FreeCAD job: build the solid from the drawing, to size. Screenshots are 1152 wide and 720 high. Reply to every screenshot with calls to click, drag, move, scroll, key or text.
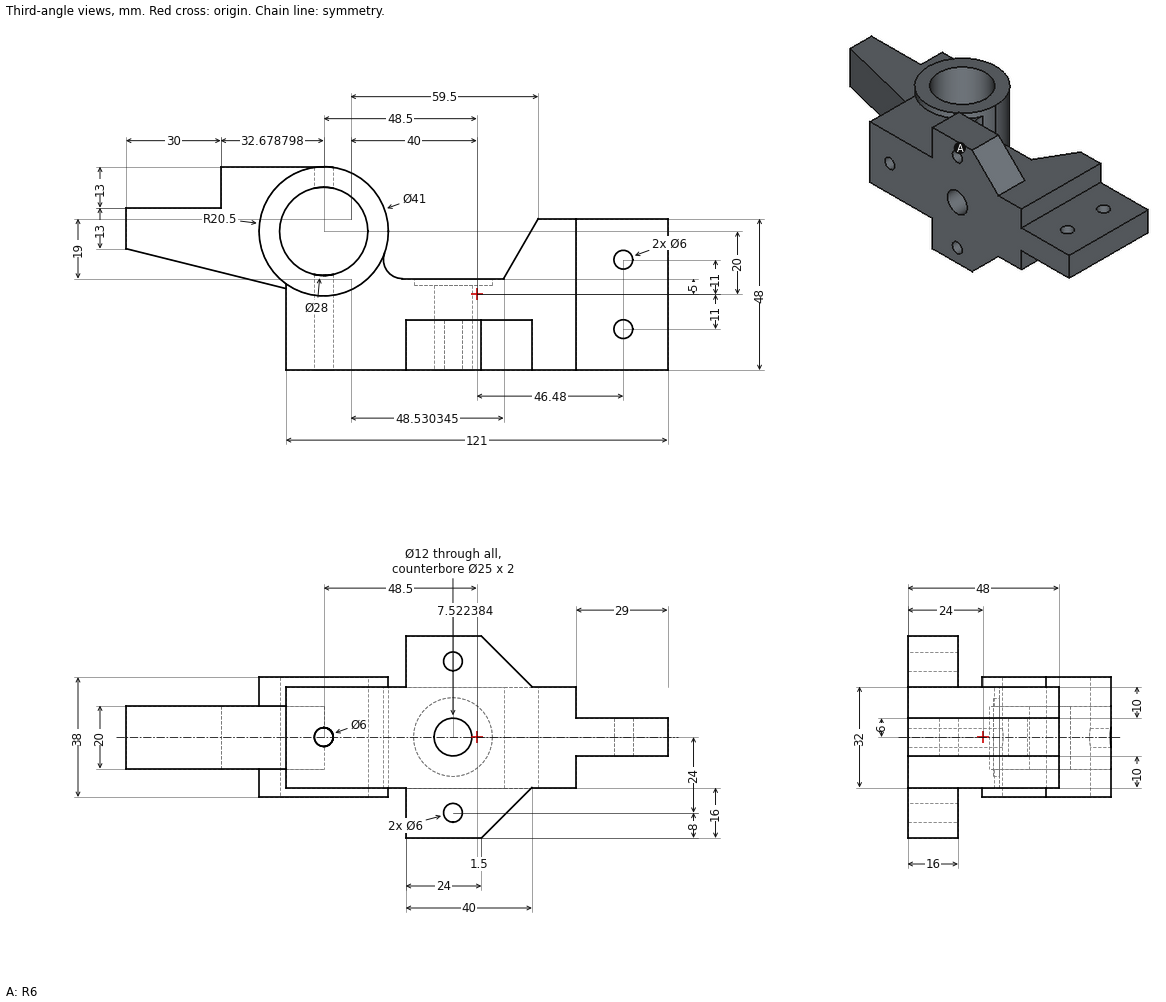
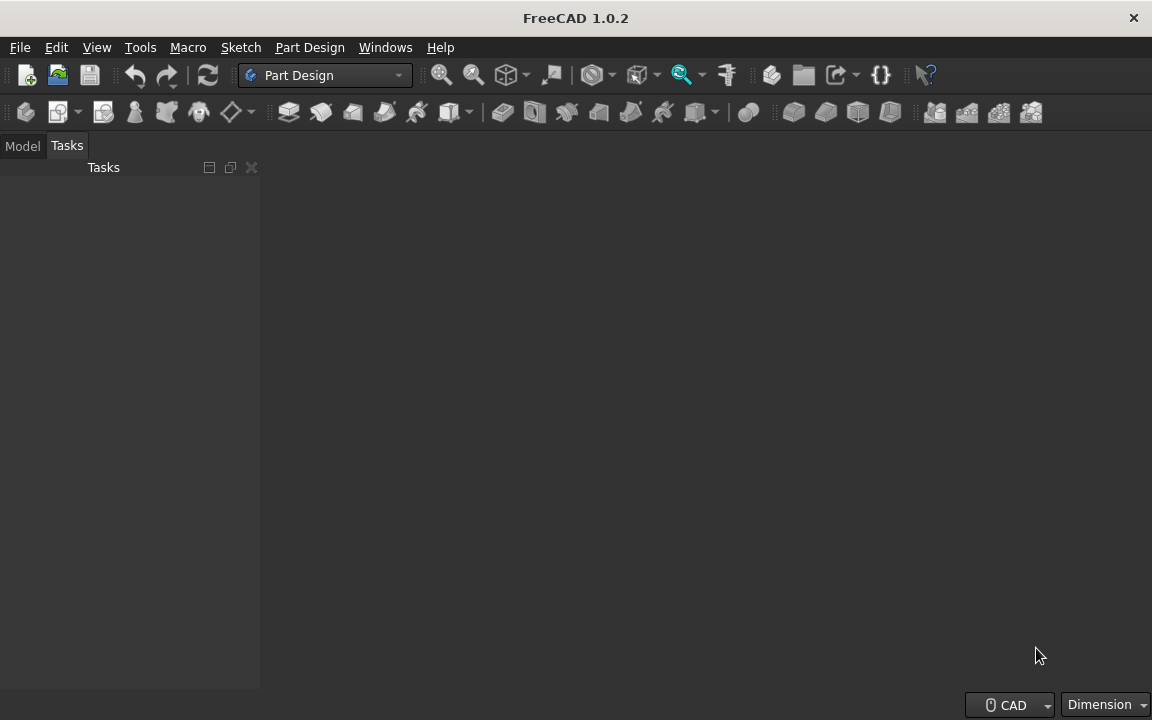
key(ctrl+n)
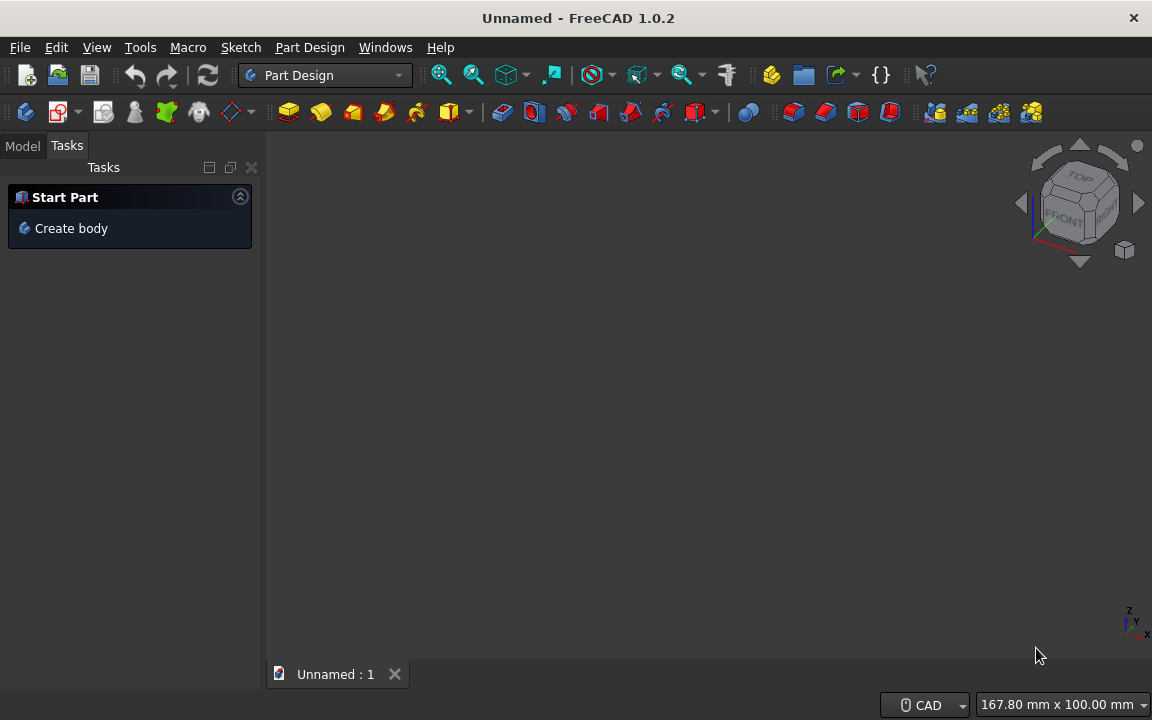
click(58, 112)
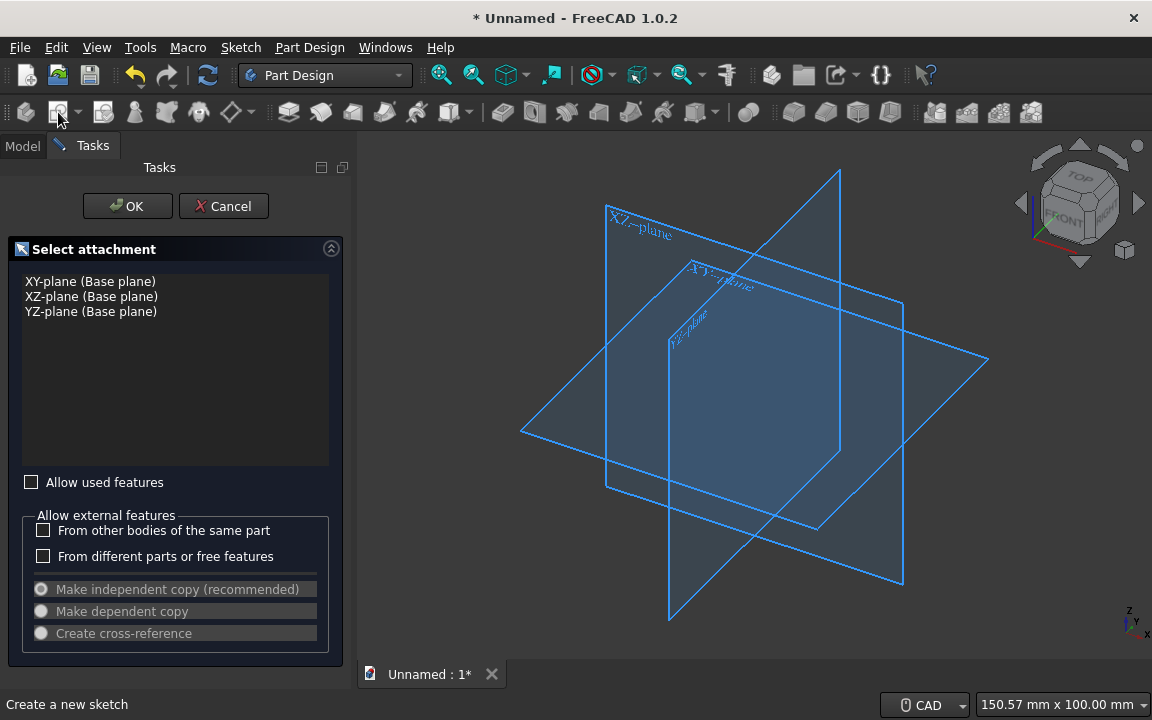
click(82, 282)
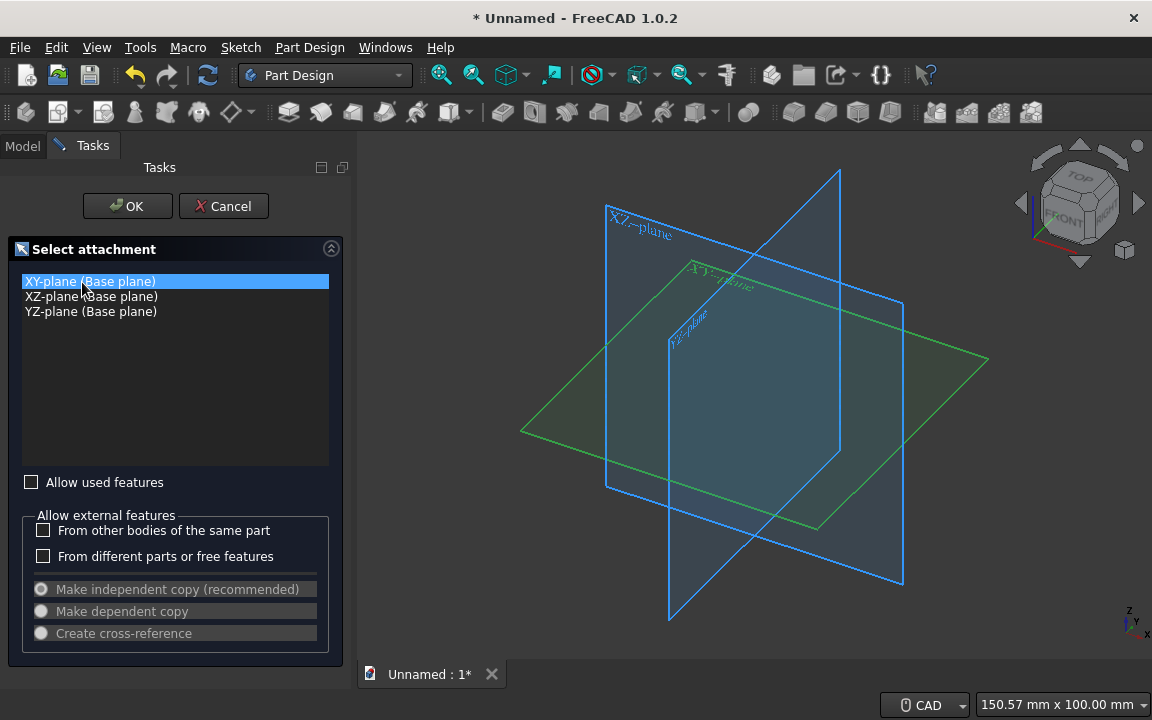
click(128, 206)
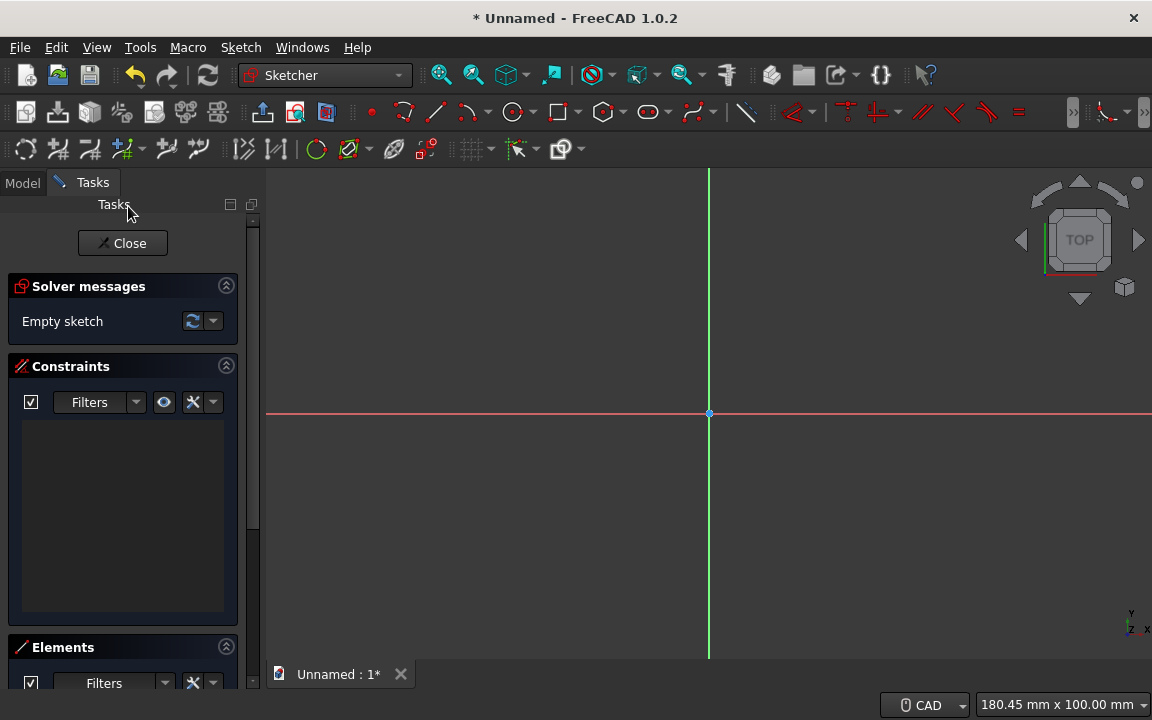
scroll(331, 413, down, 1)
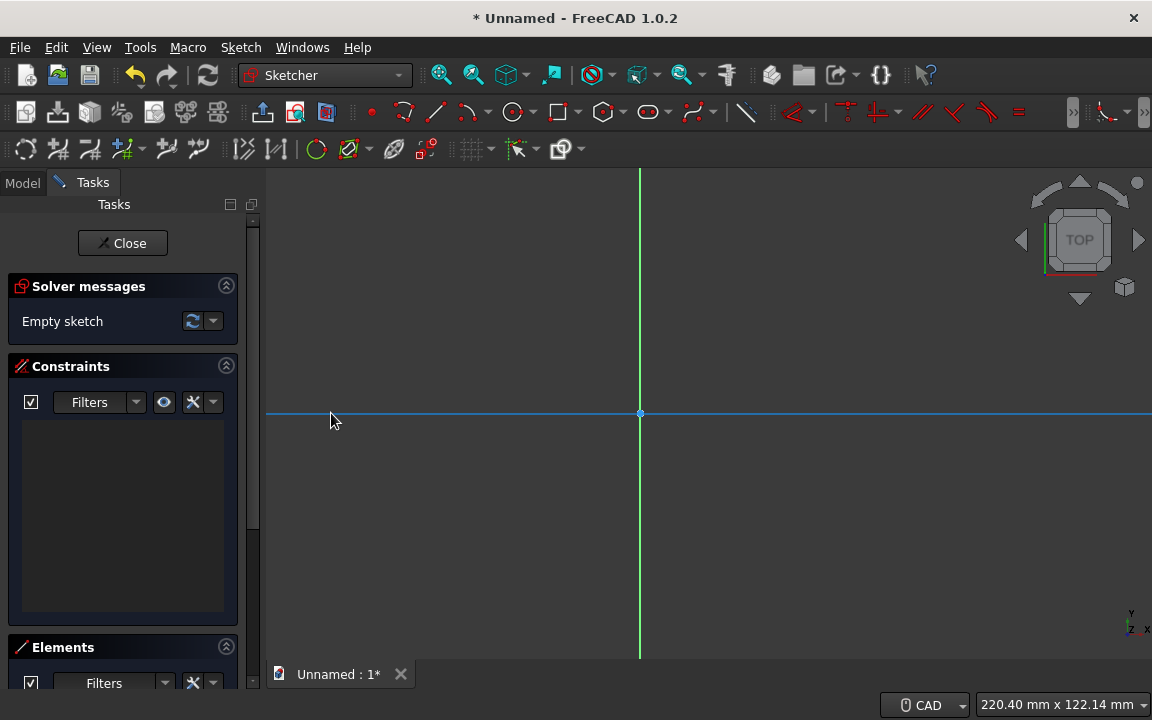
key(g)
key(v)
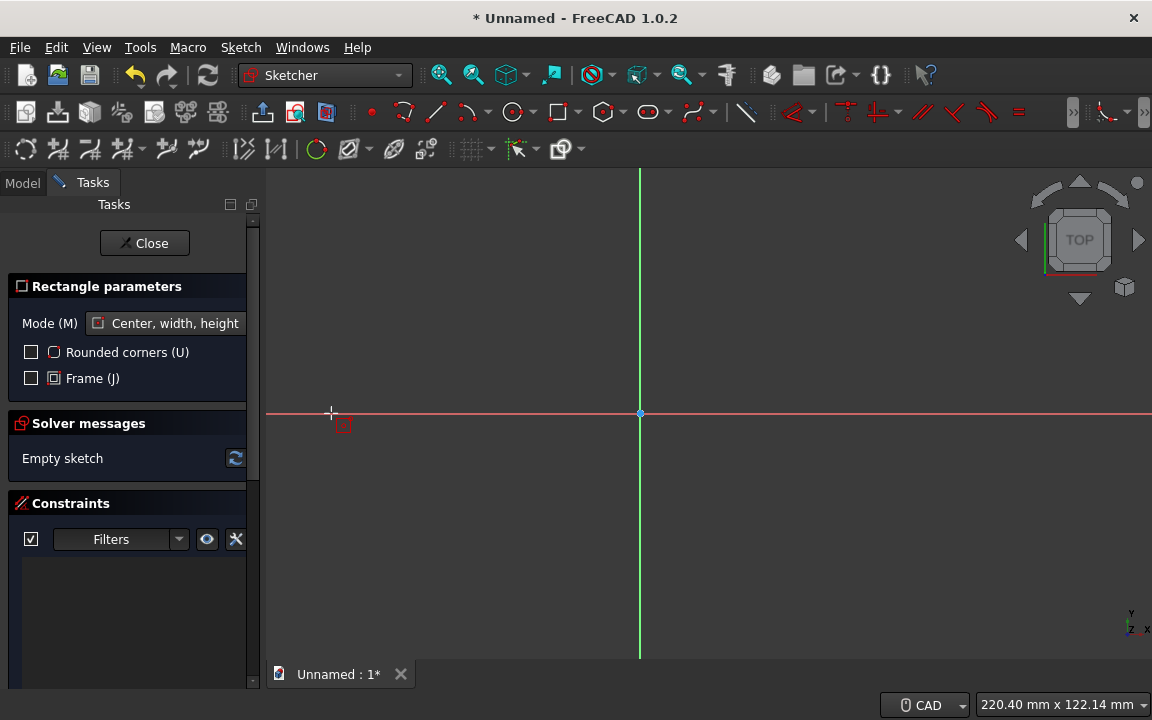
click(640, 414)
move(884, 317)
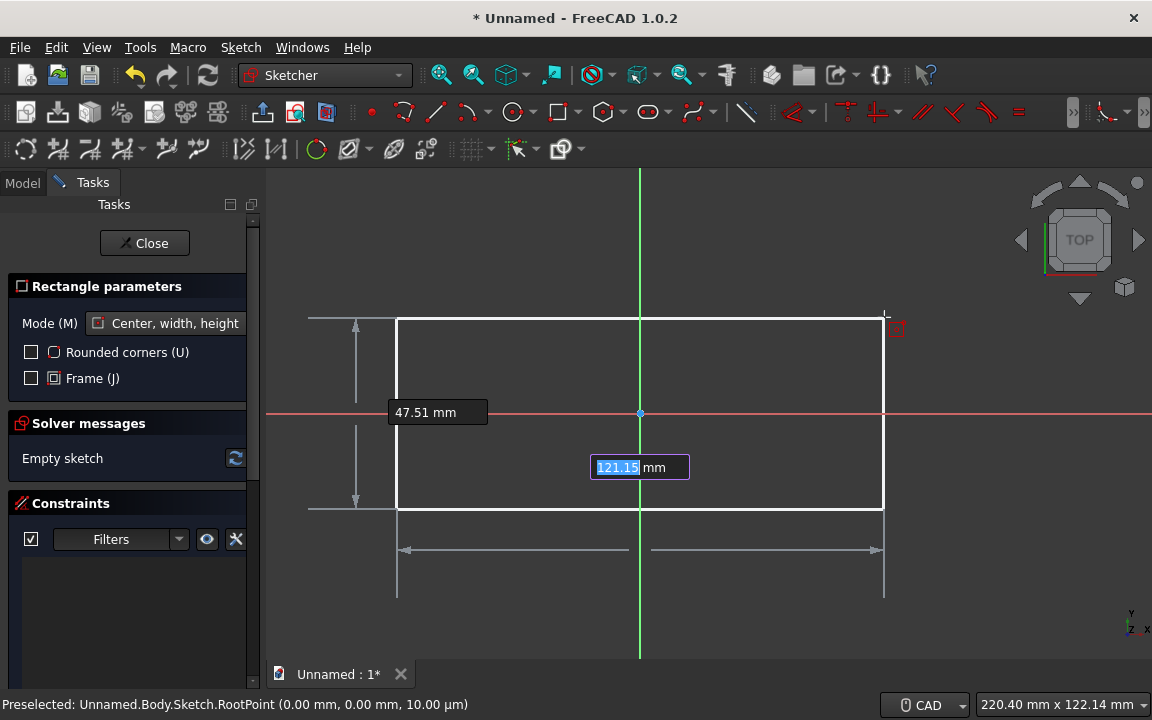
text(121)
key(Tab)
text(48)
key(Return)
key(Escape)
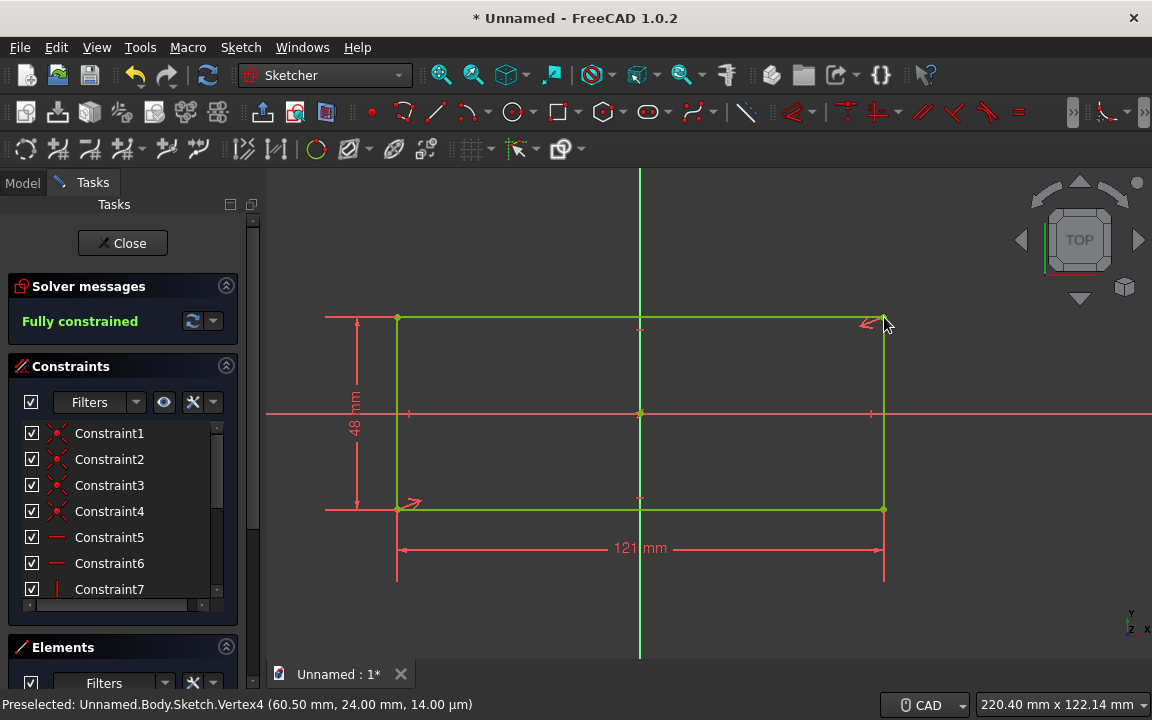
click(123, 243)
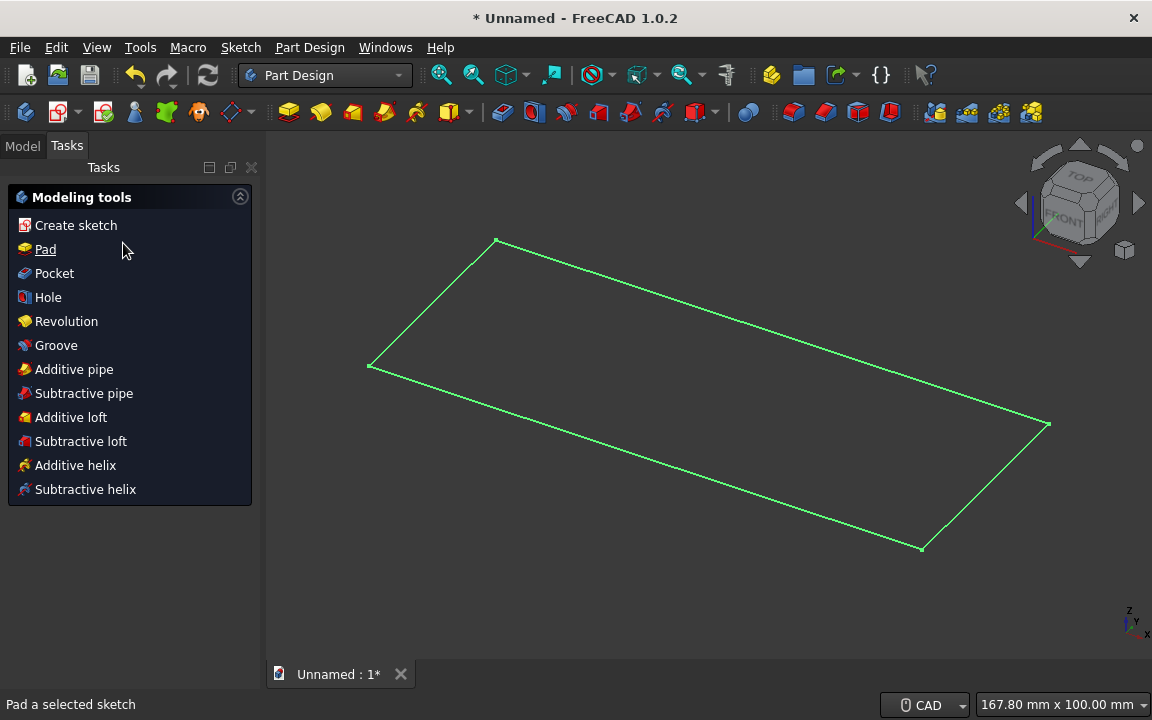
click(290, 112)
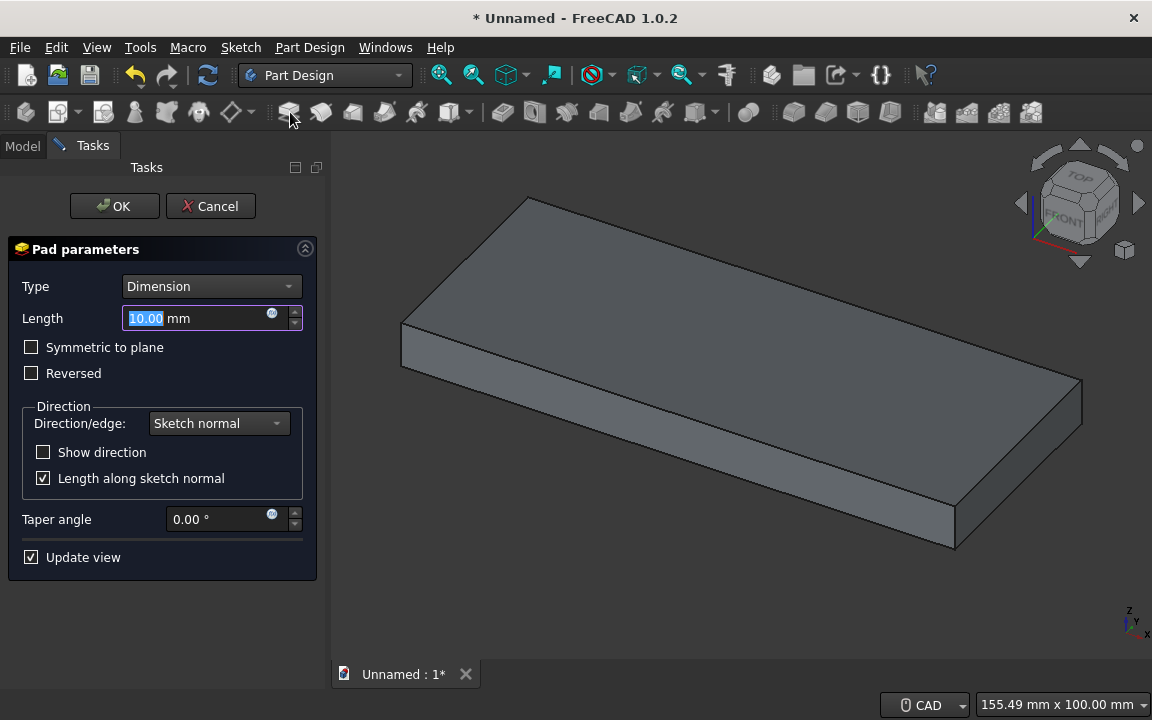
text(32)
key(Tab)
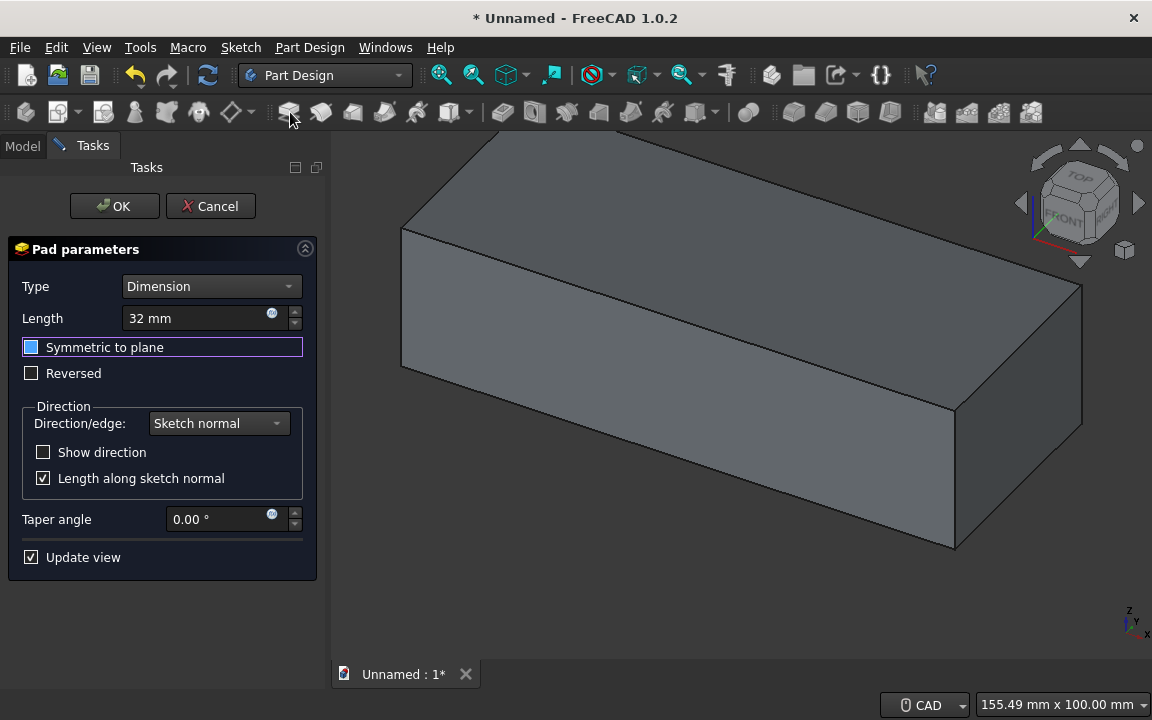
click(30, 347)